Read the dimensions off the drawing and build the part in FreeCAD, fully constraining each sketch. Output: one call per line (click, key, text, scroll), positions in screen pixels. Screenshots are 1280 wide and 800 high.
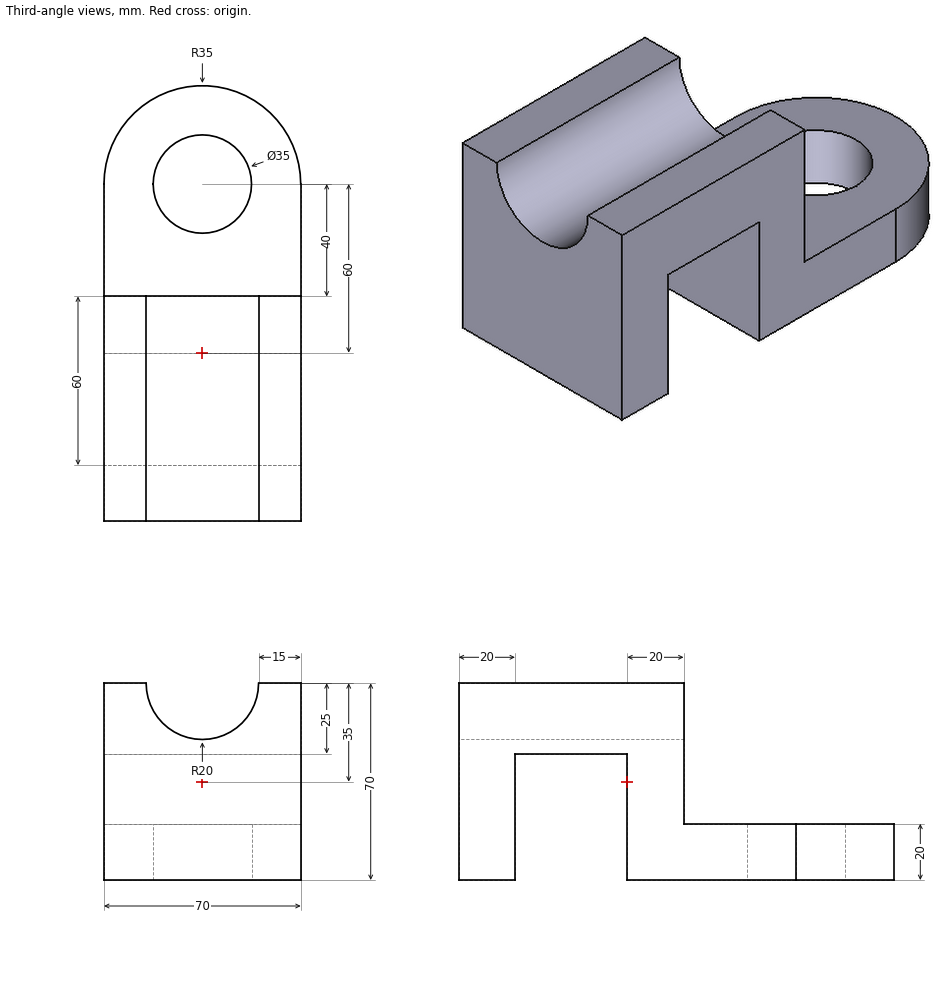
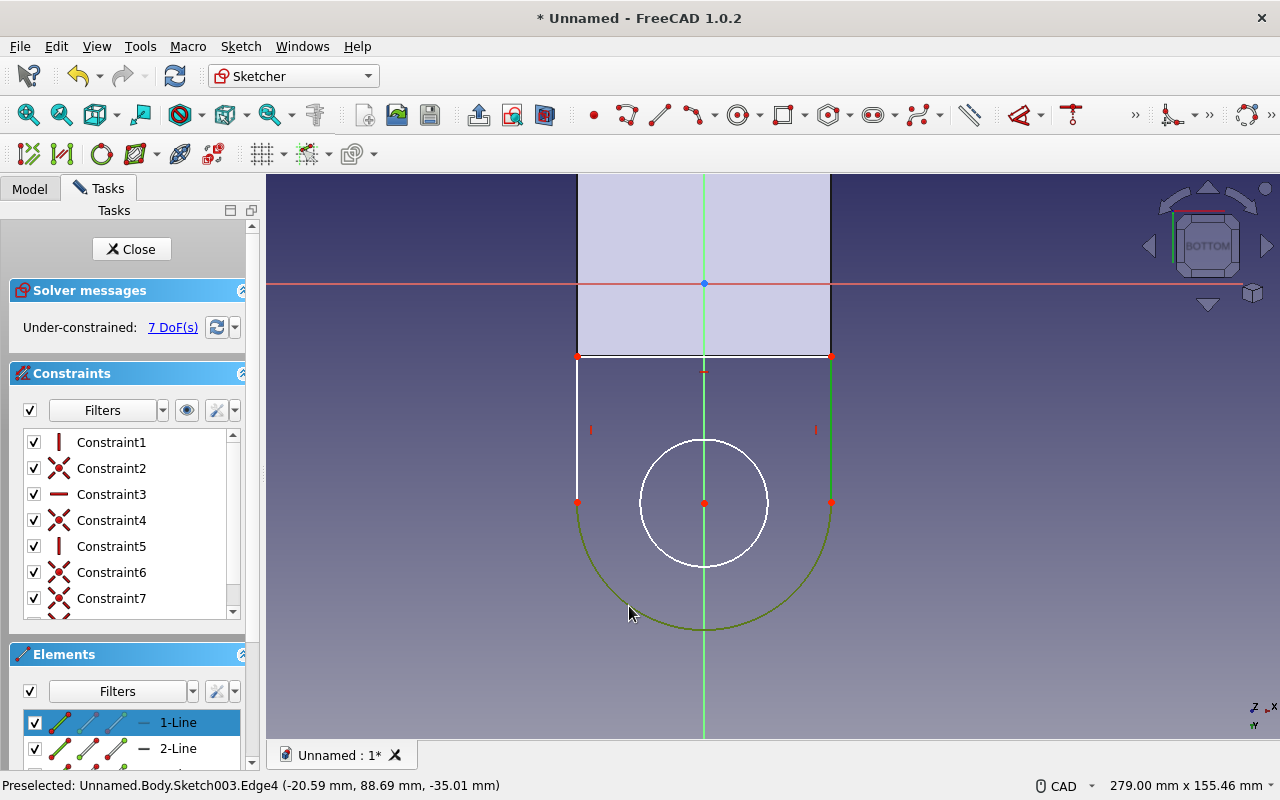
key(t)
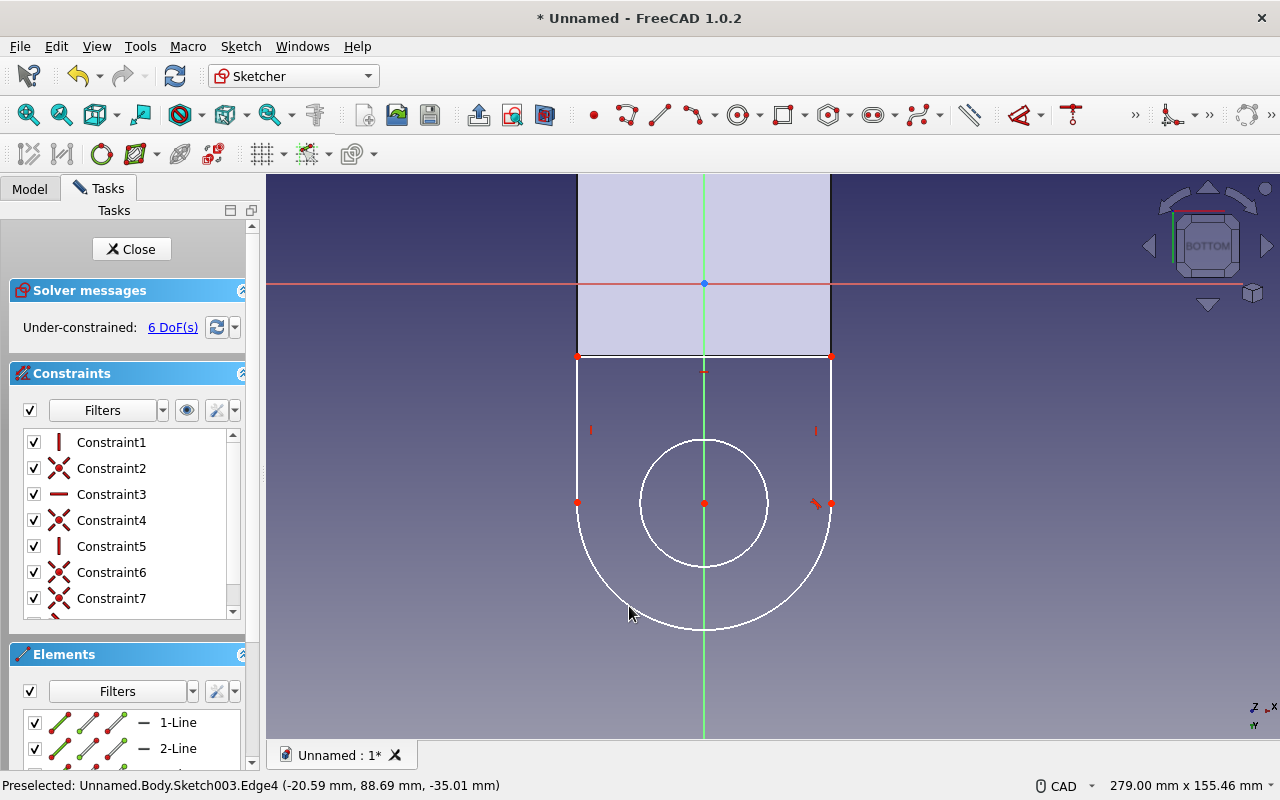
click(577, 401)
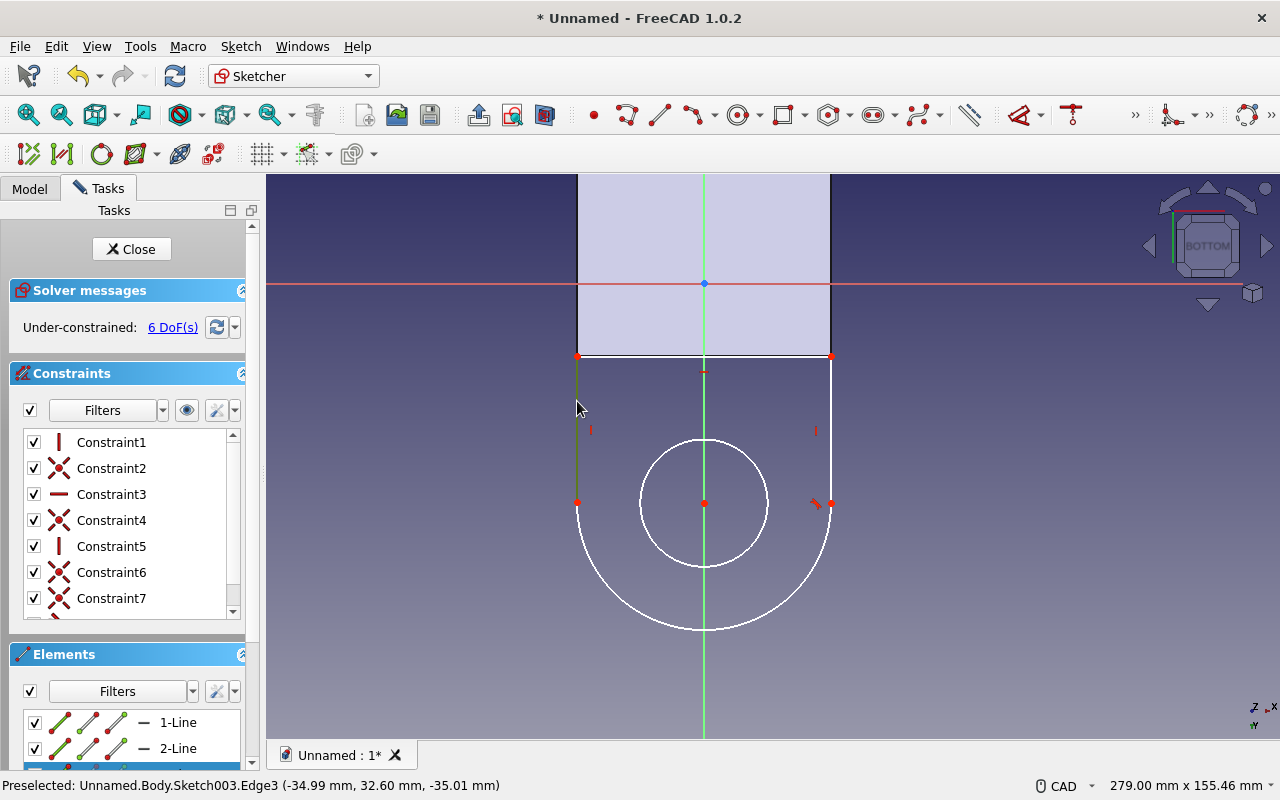
click(629, 606)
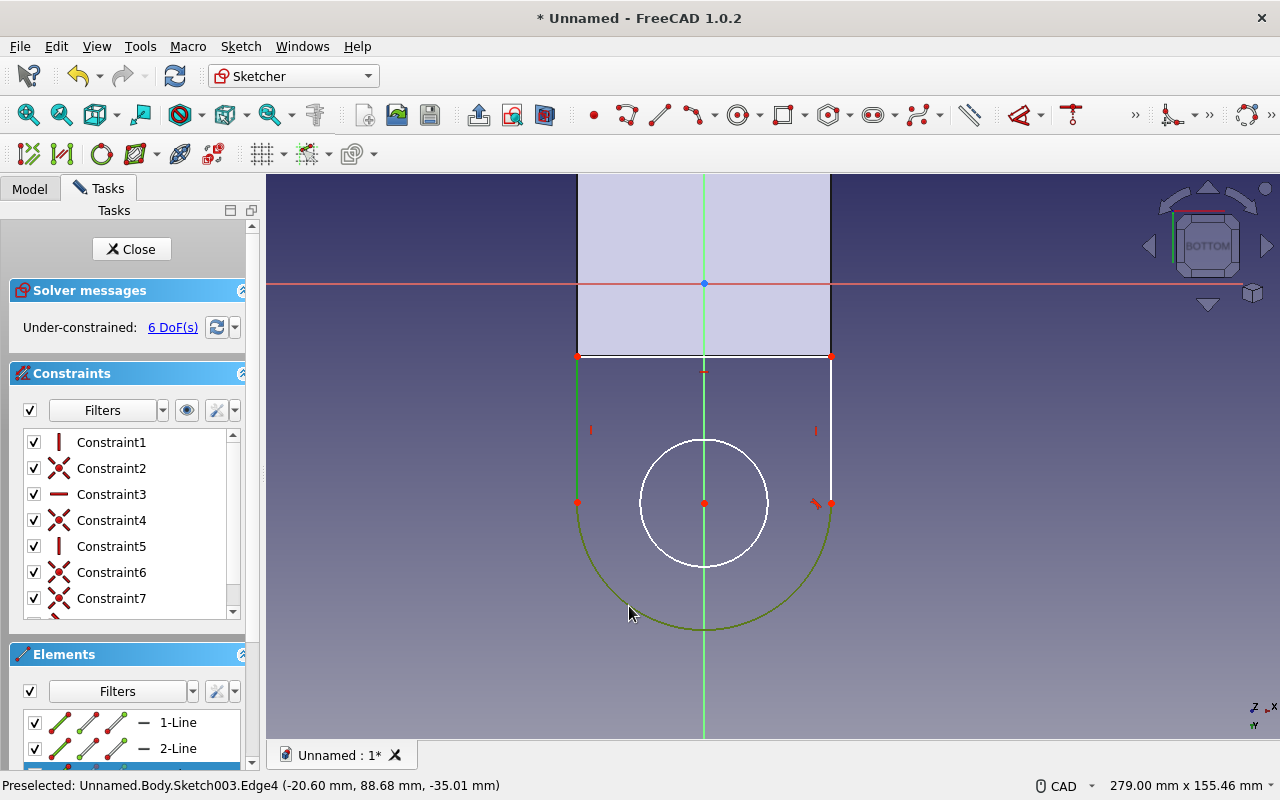
key(t)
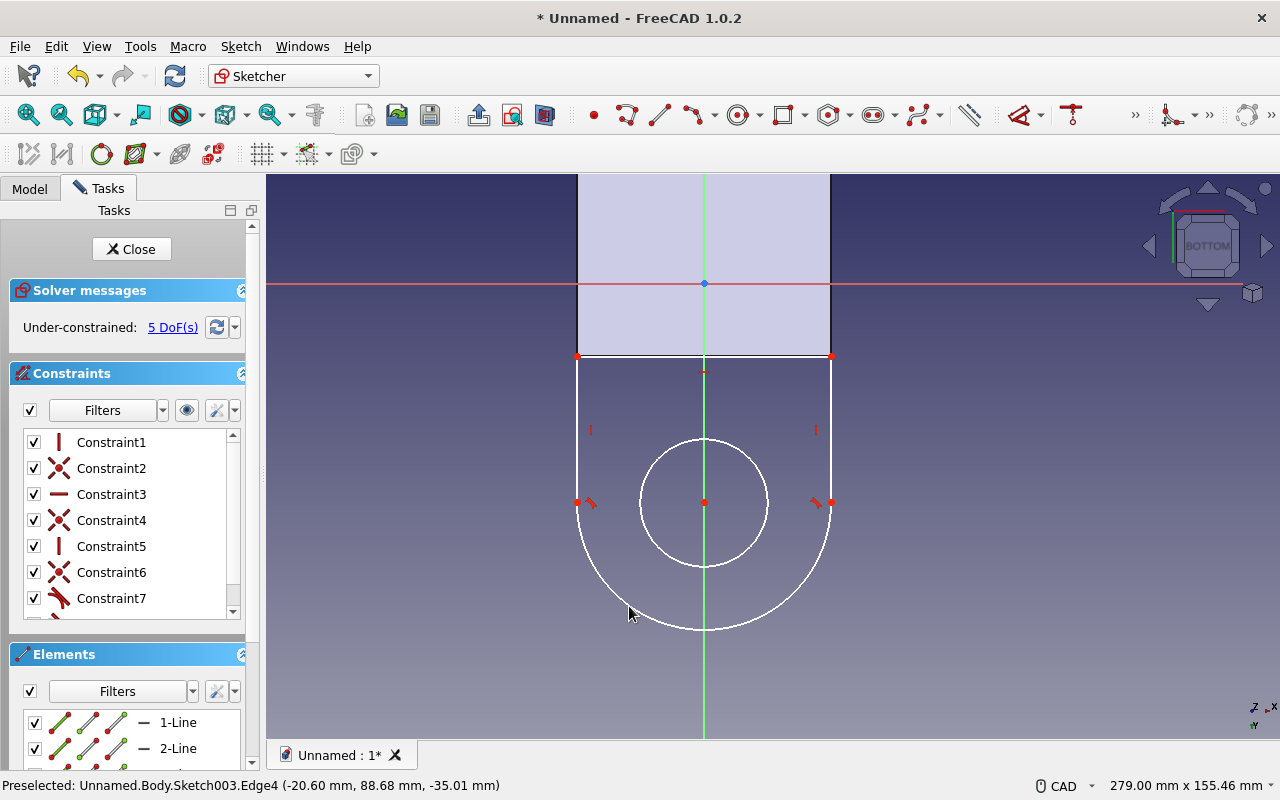
click(704, 503)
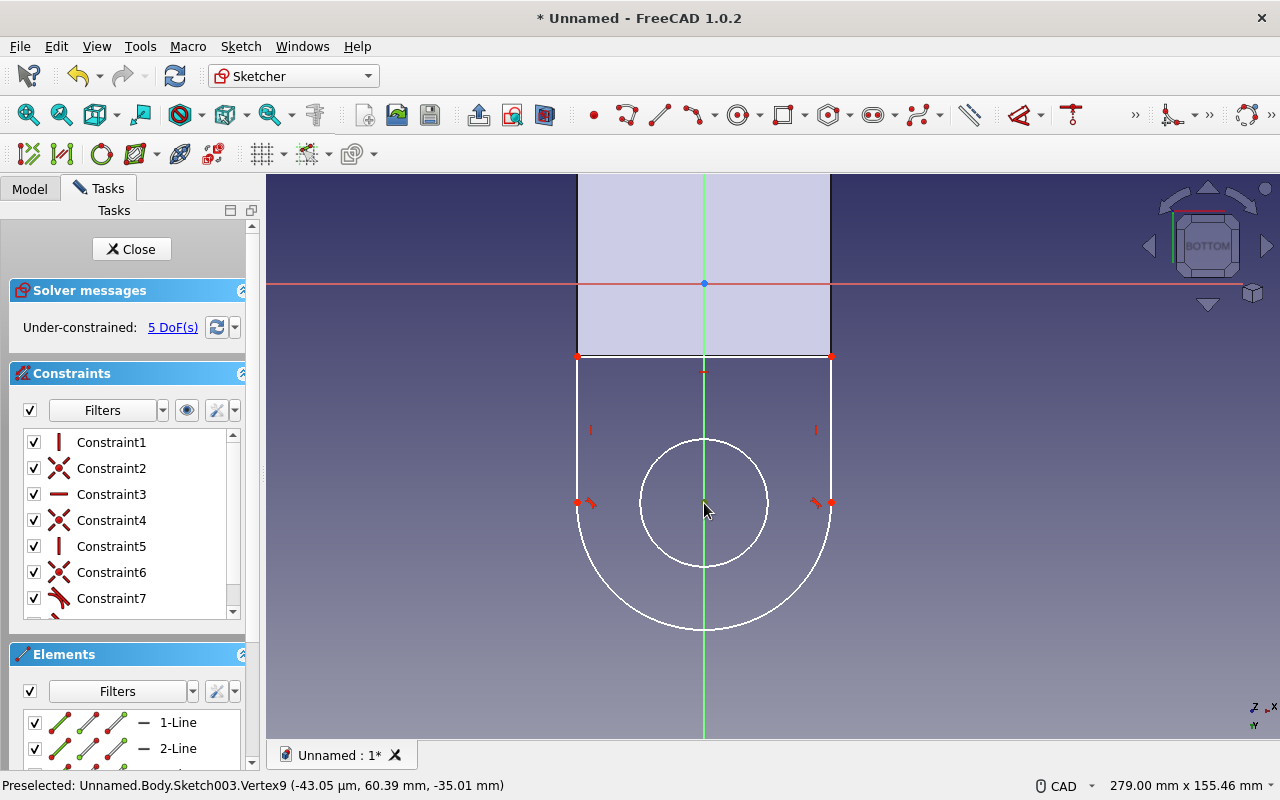
click(704, 675)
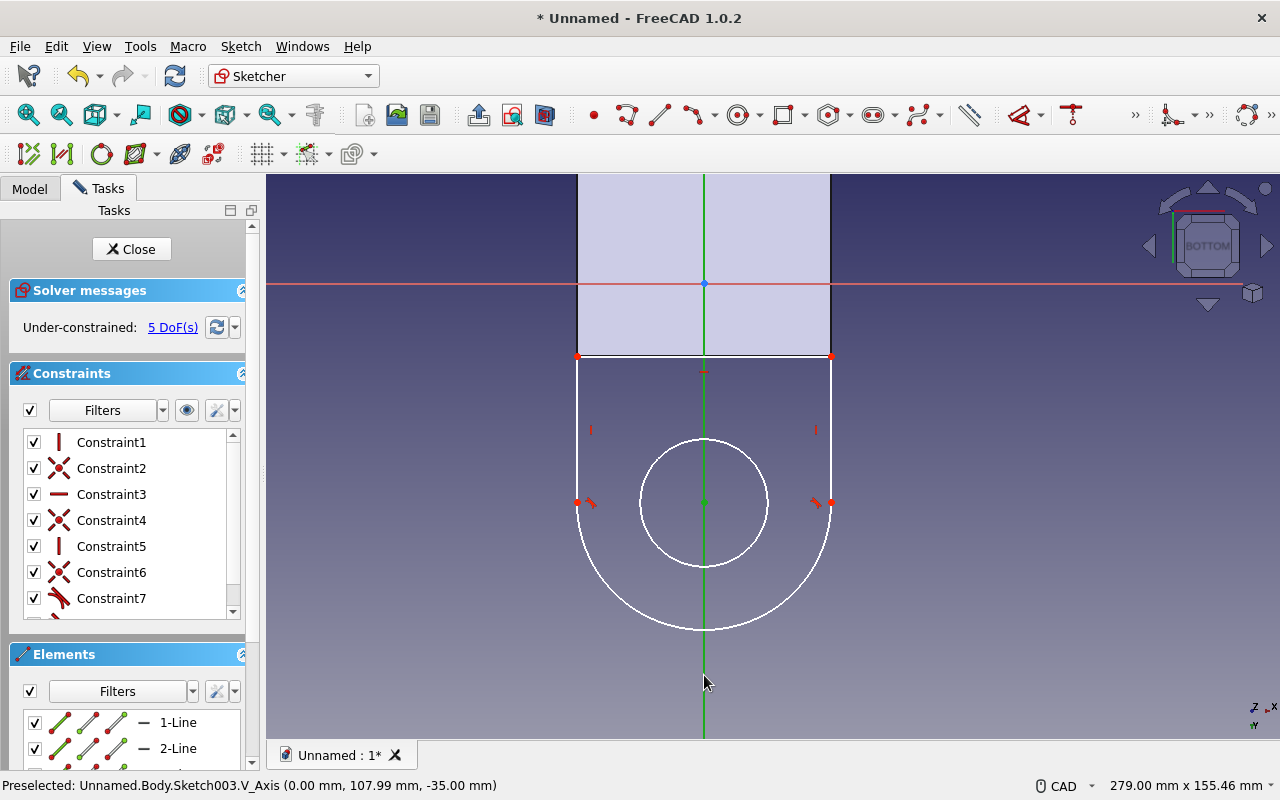
click(1071, 116)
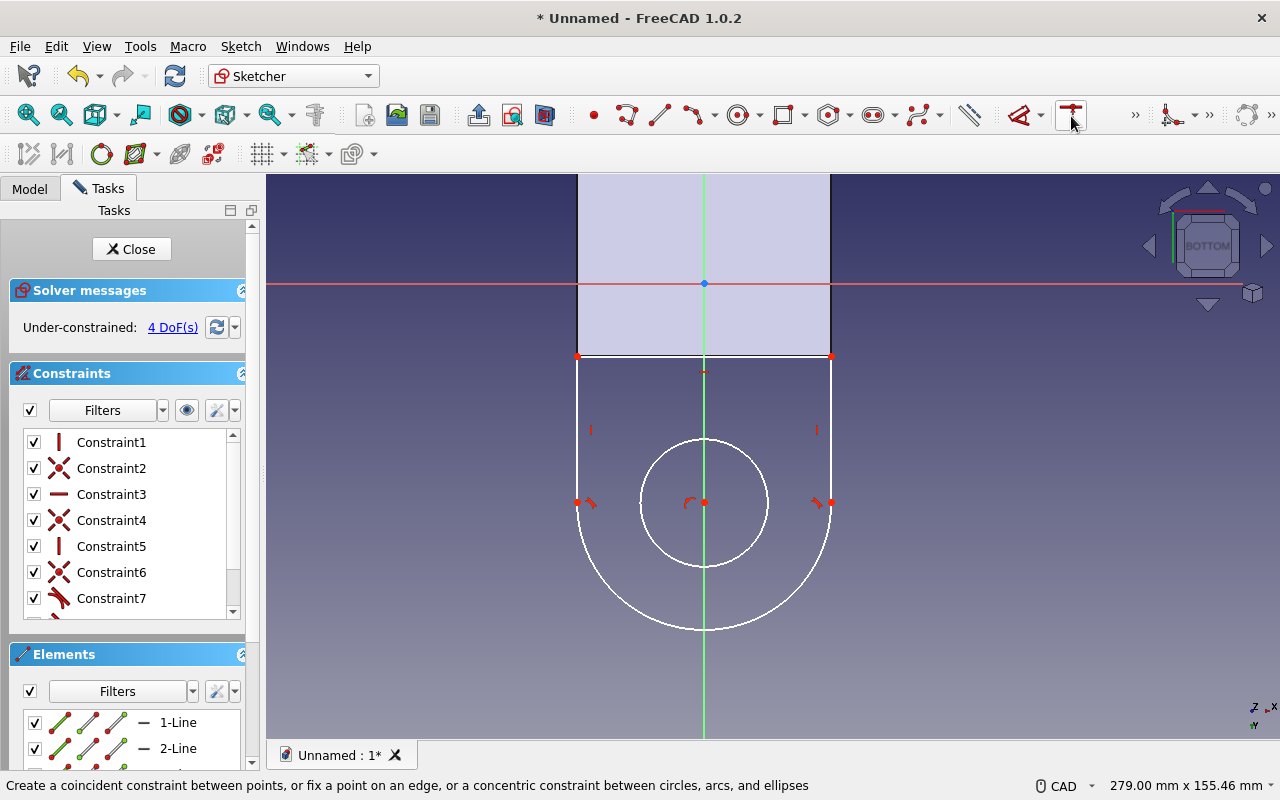
click(1018, 116)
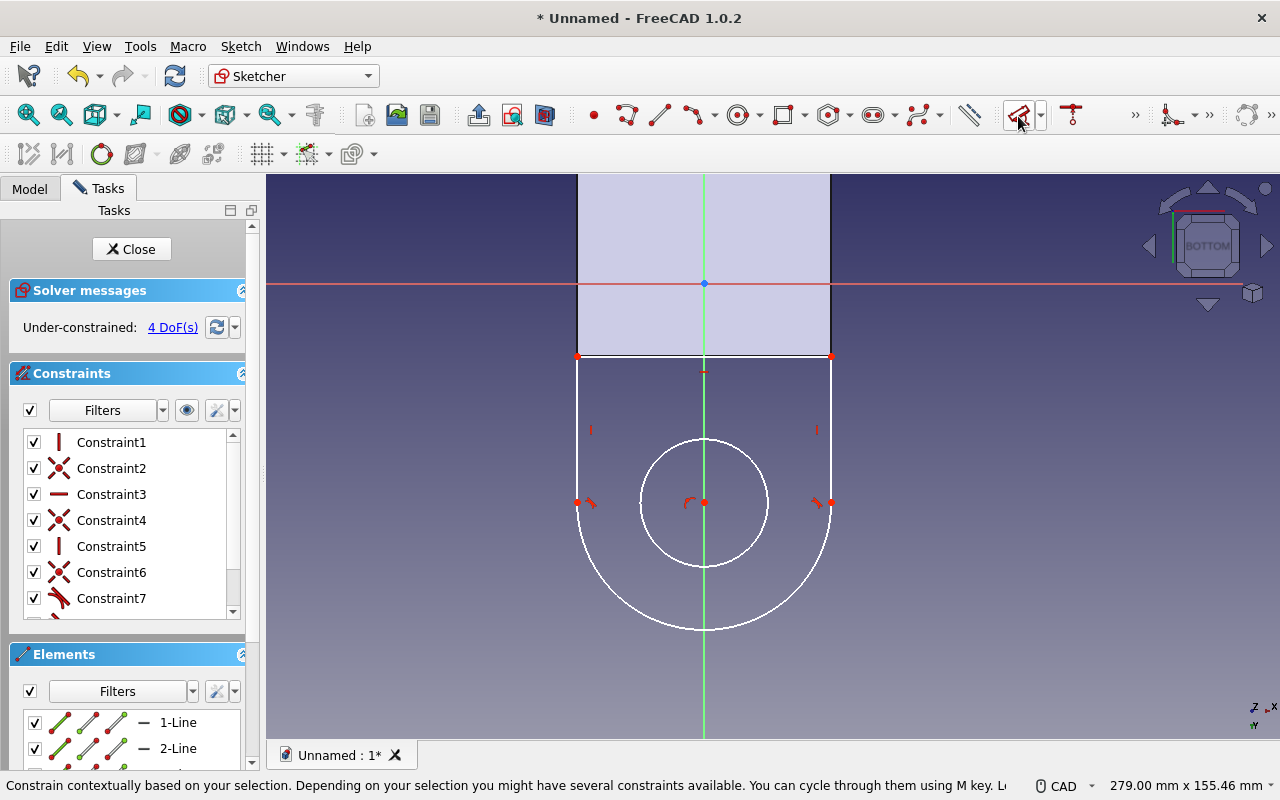
click(630, 606)
click(611, 632)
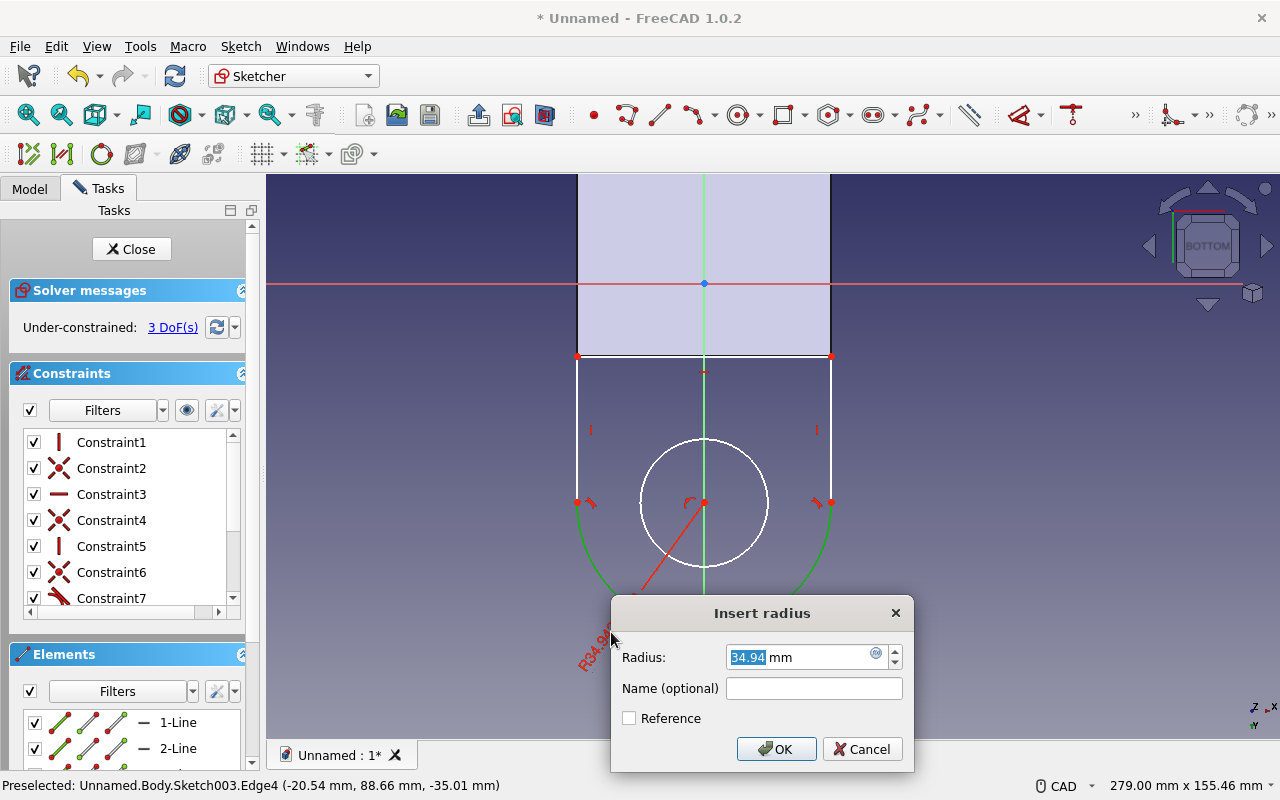
text(35)
key(Return)